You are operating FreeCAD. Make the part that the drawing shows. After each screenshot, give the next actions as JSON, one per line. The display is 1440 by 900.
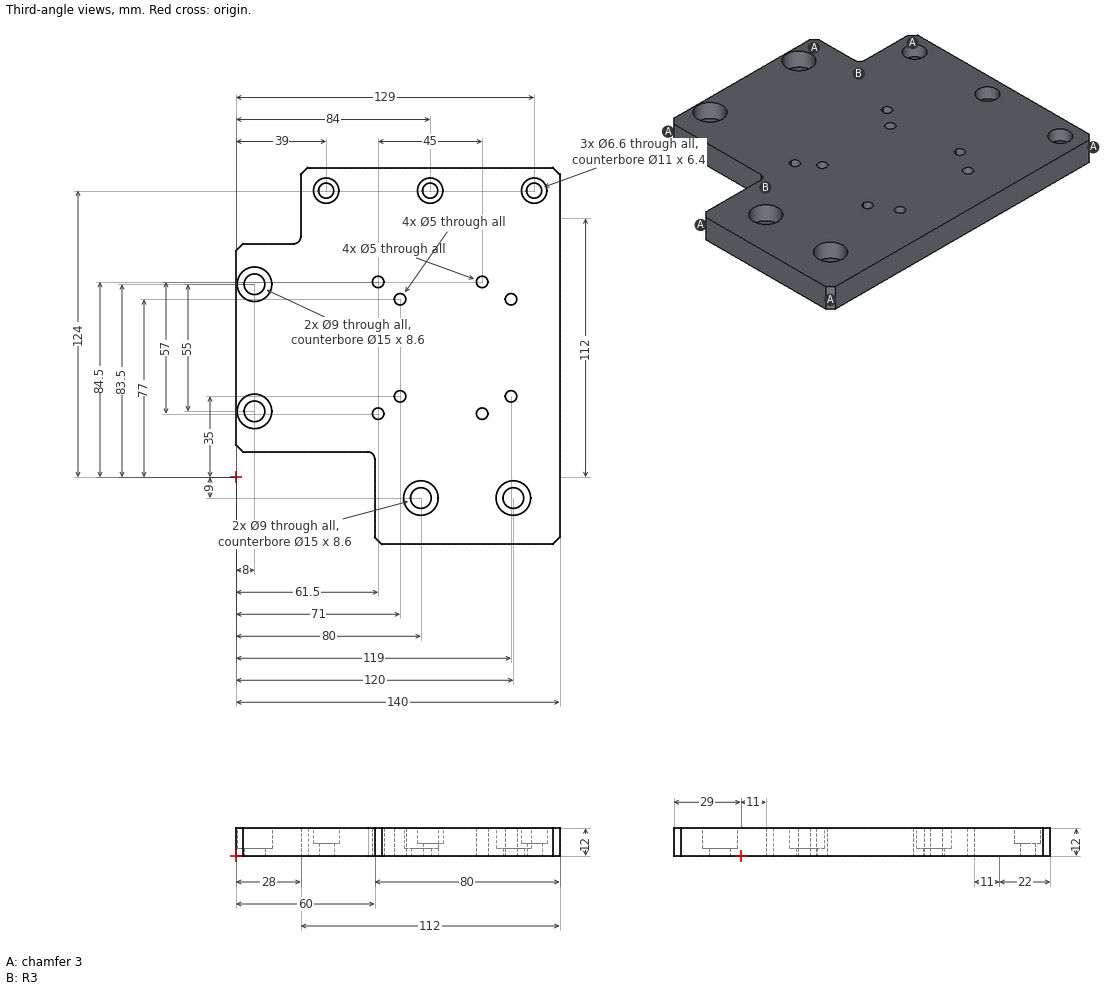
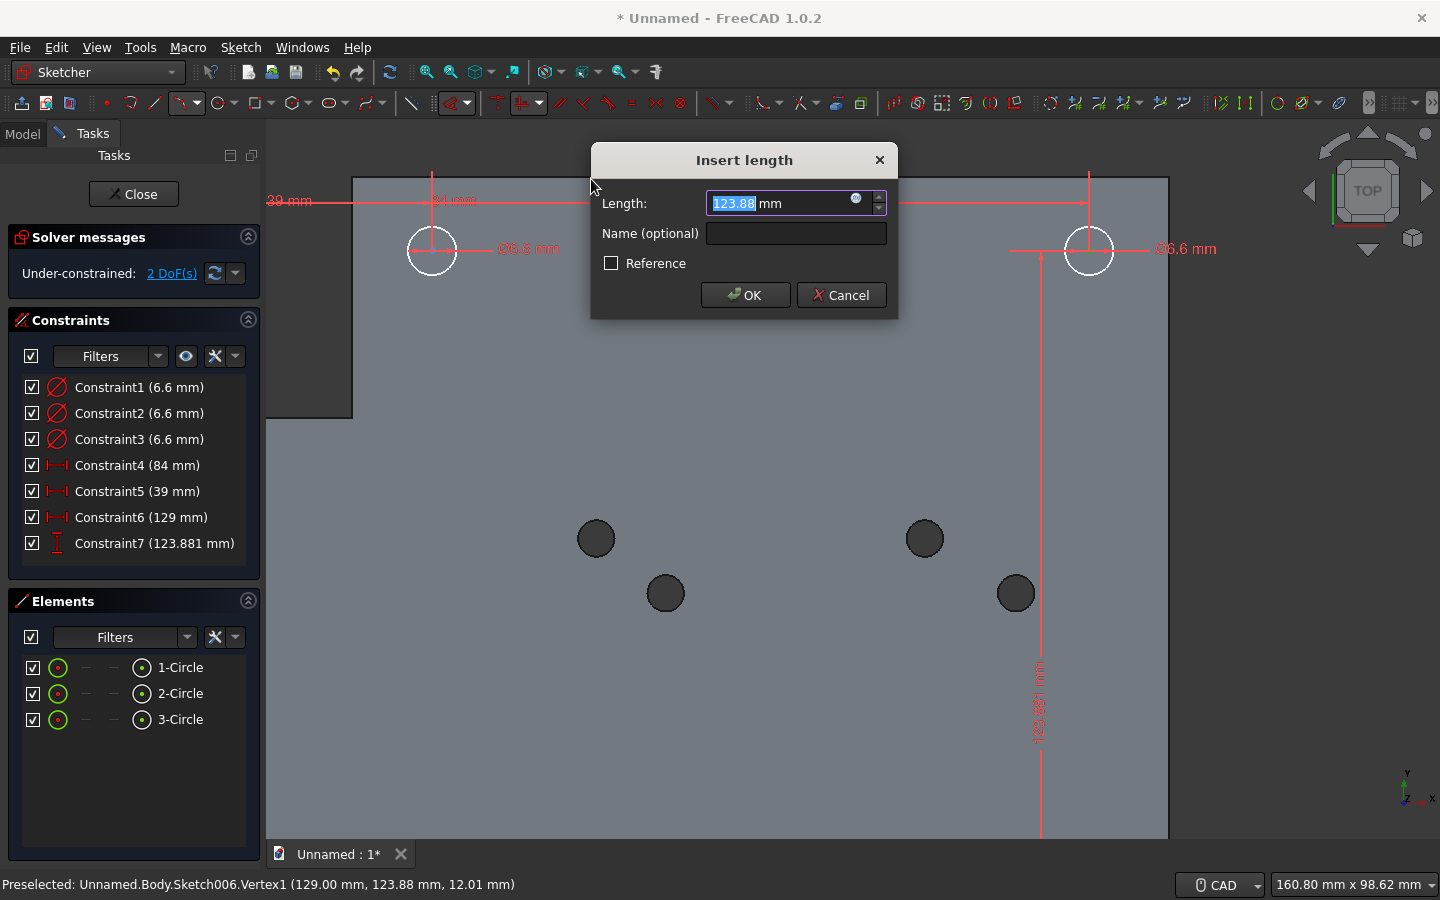
{"action": "type", "text": "124"}
{"action": "key", "text": "Return"}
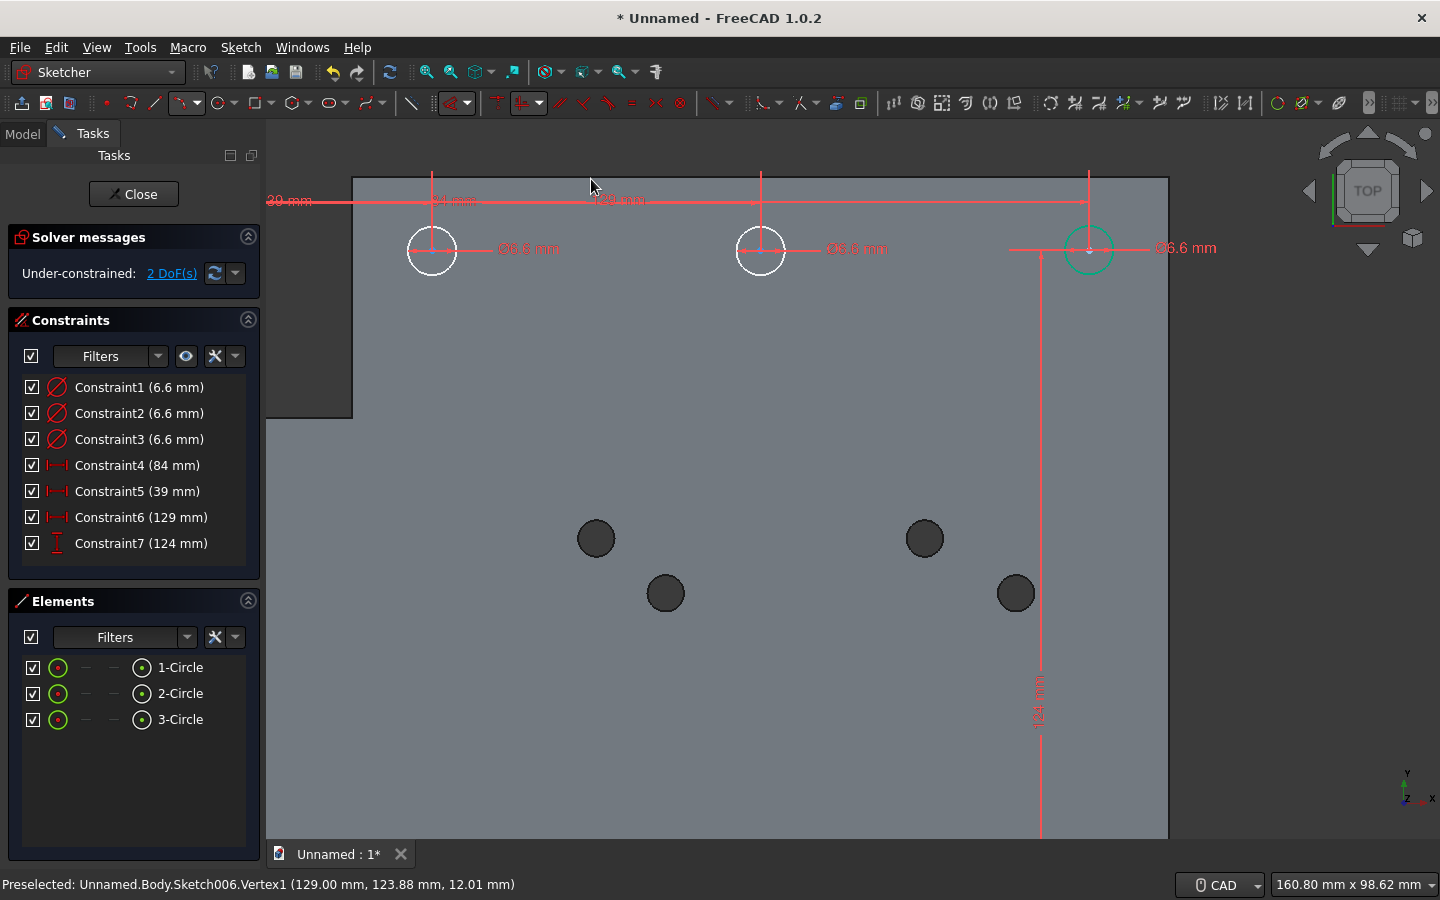
{"action": "left_click", "coordinate": [761, 251]}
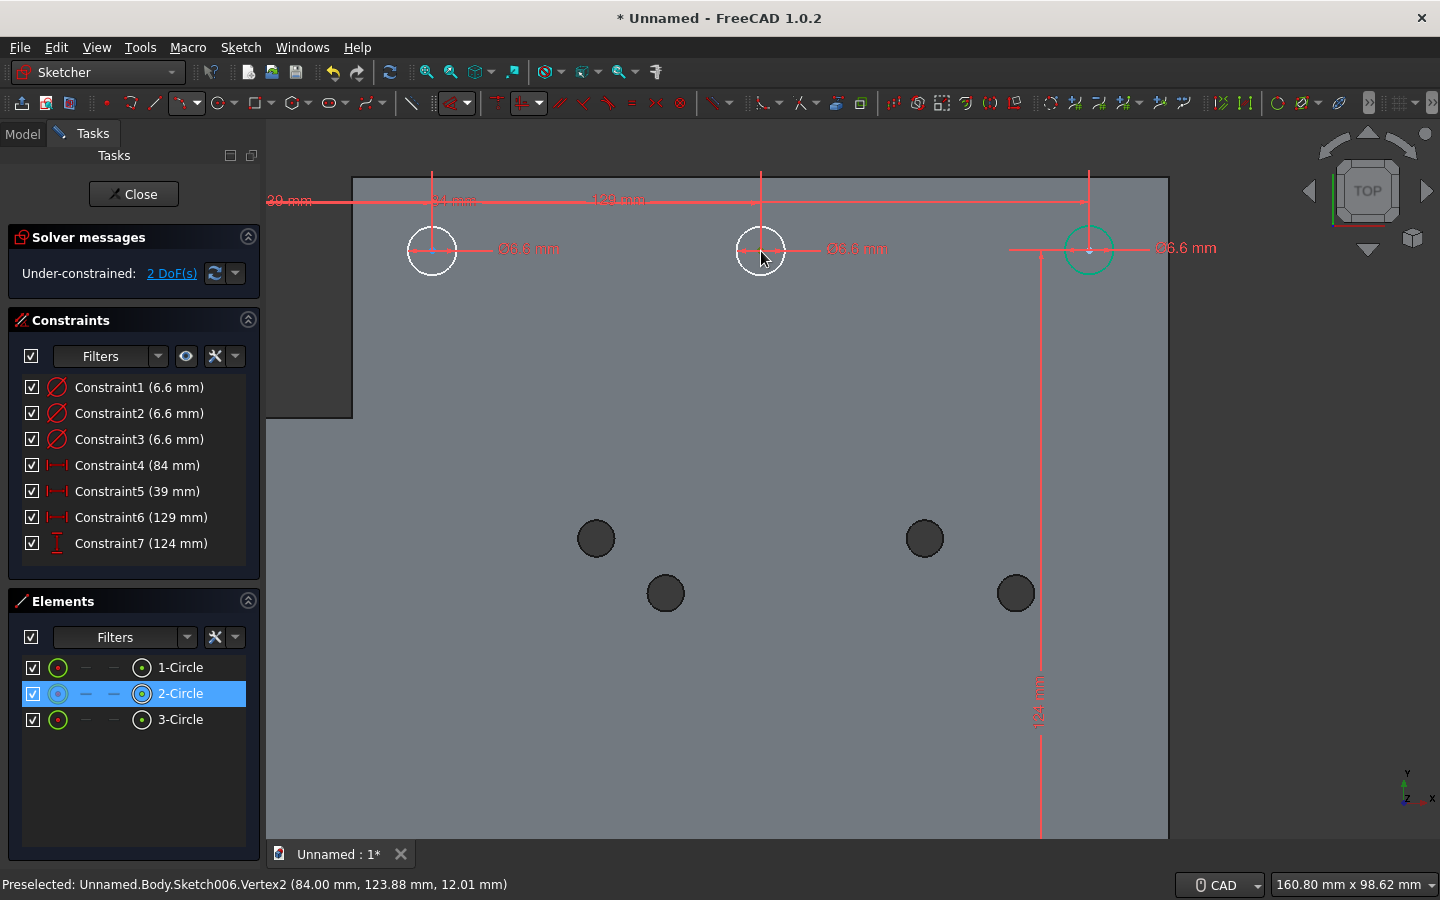
{"action": "key", "text": "i"}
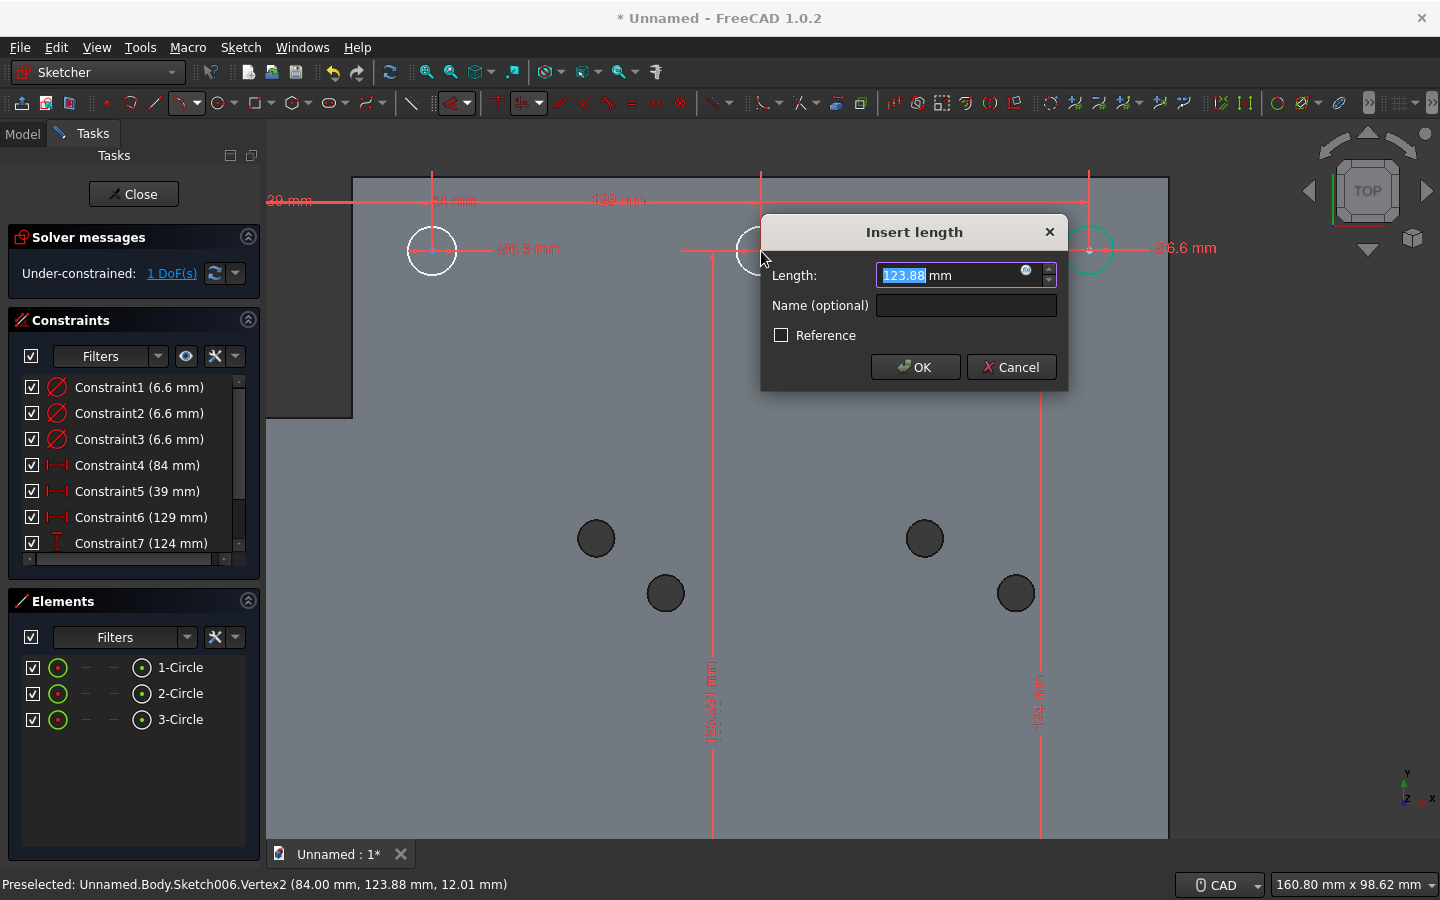
{"action": "type", "text": "124"}
{"action": "key", "text": "Return"}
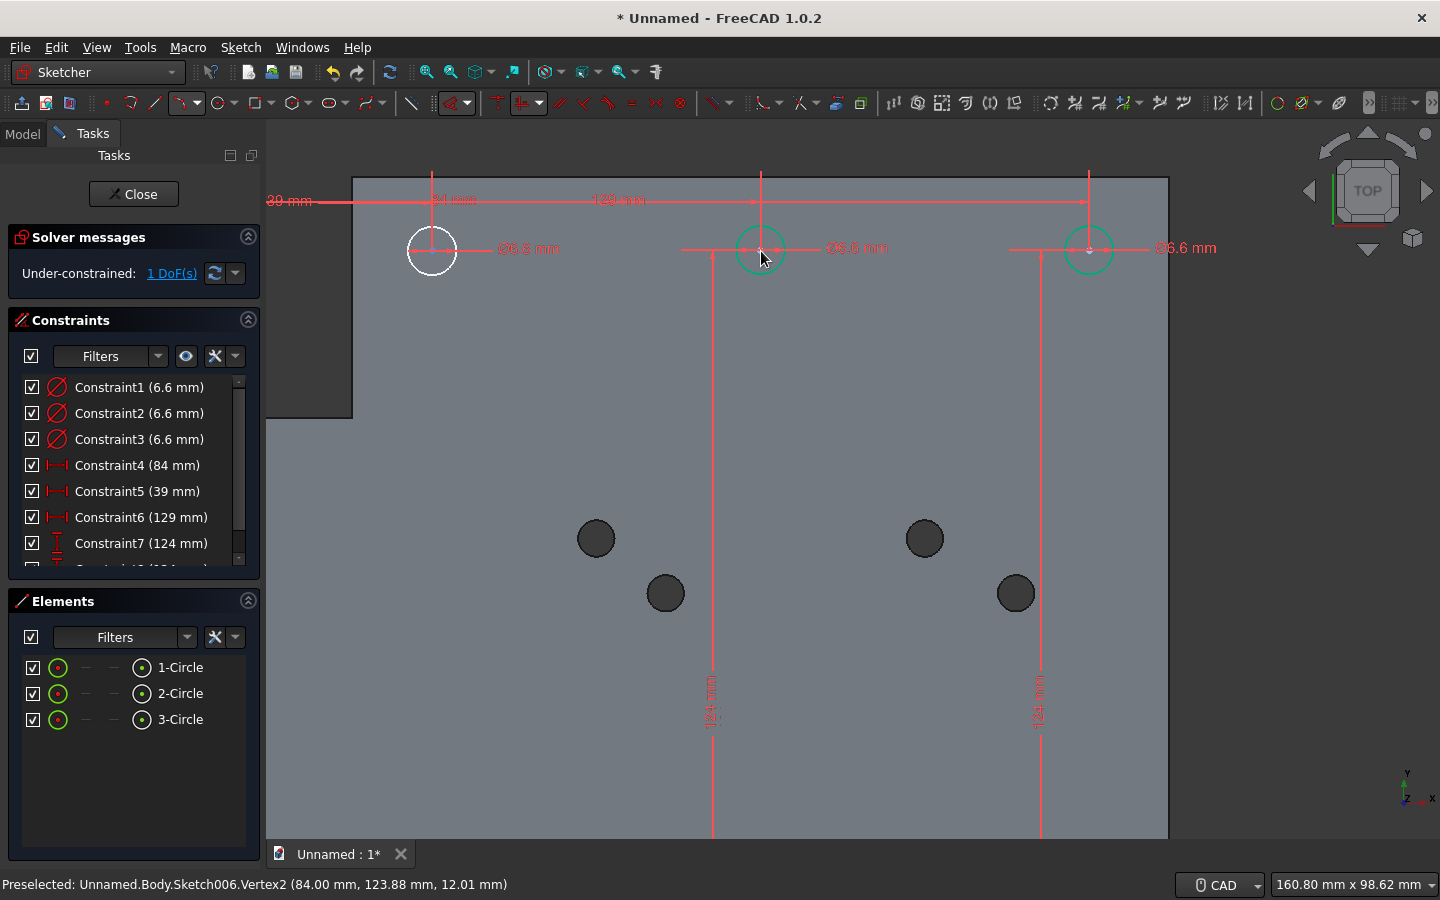
{"action": "left_click", "coordinate": [432, 251]}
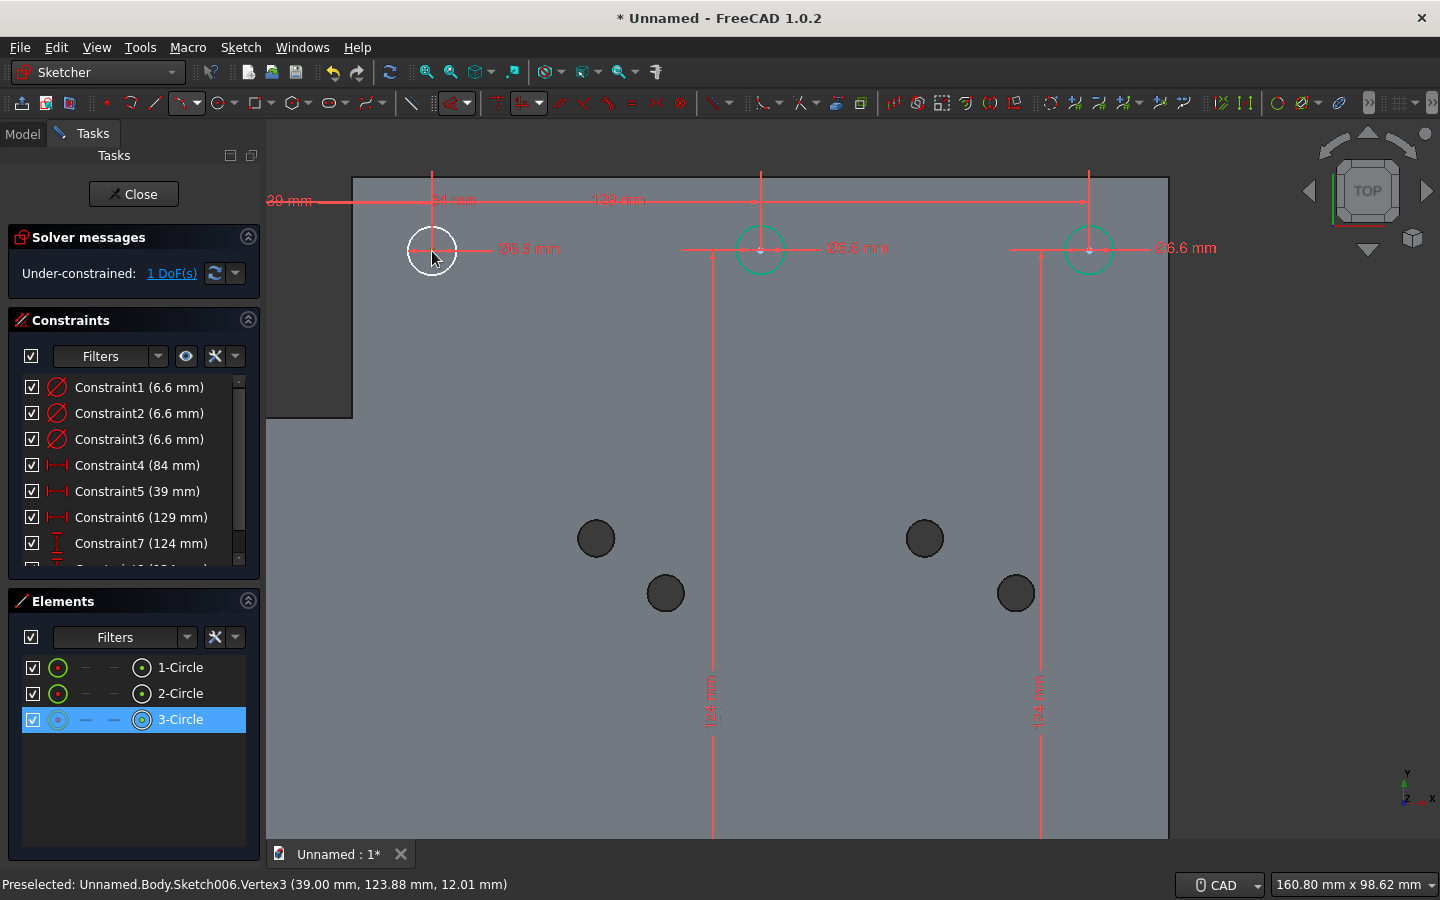
{"action": "left_click", "coordinate": [470, 104]}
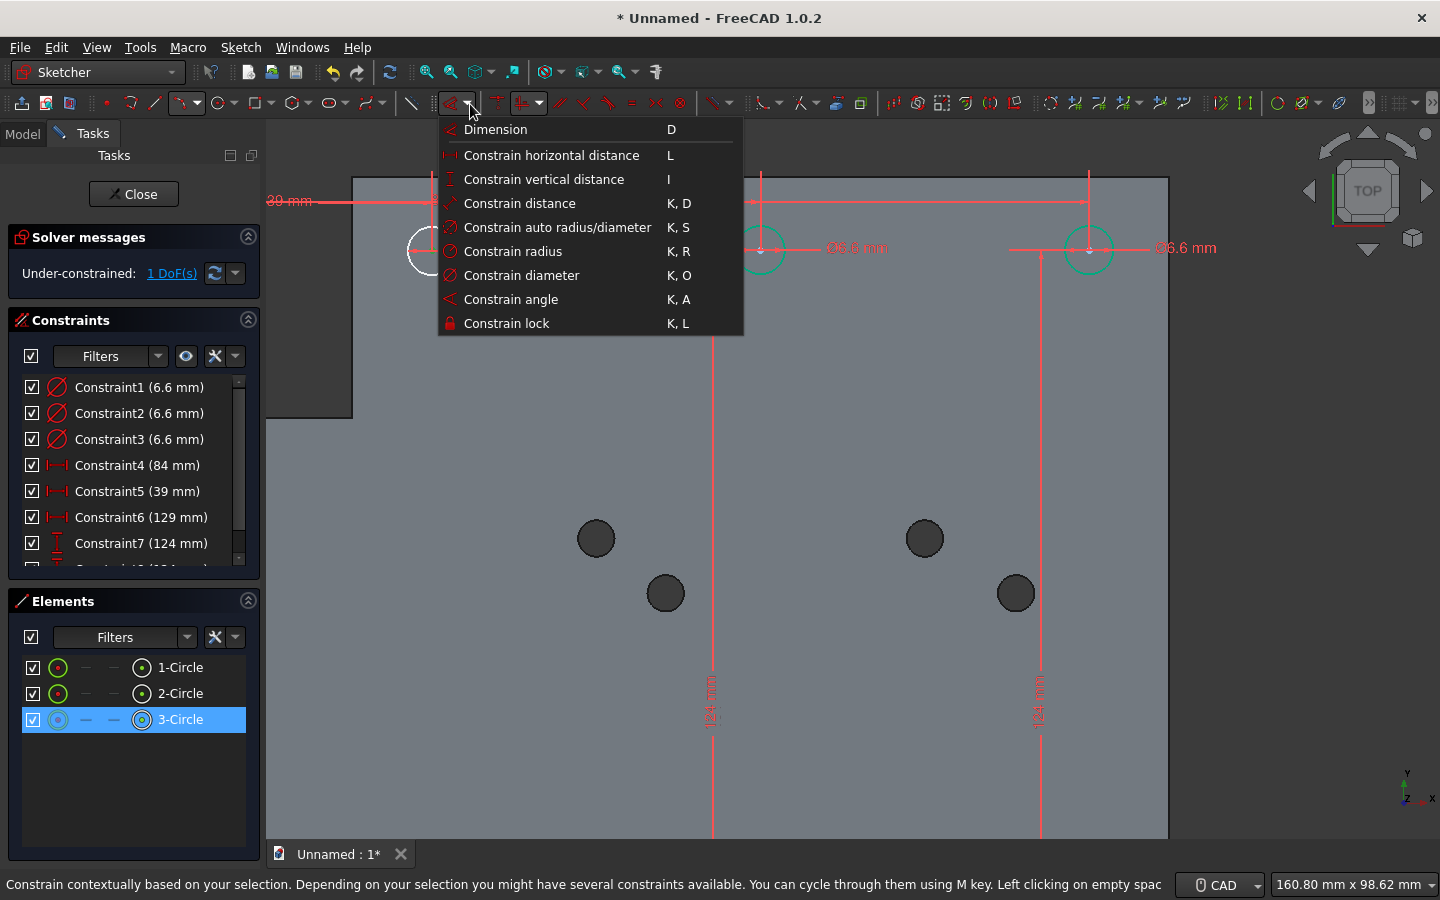
{"action": "left_click", "coordinate": [591, 179]}